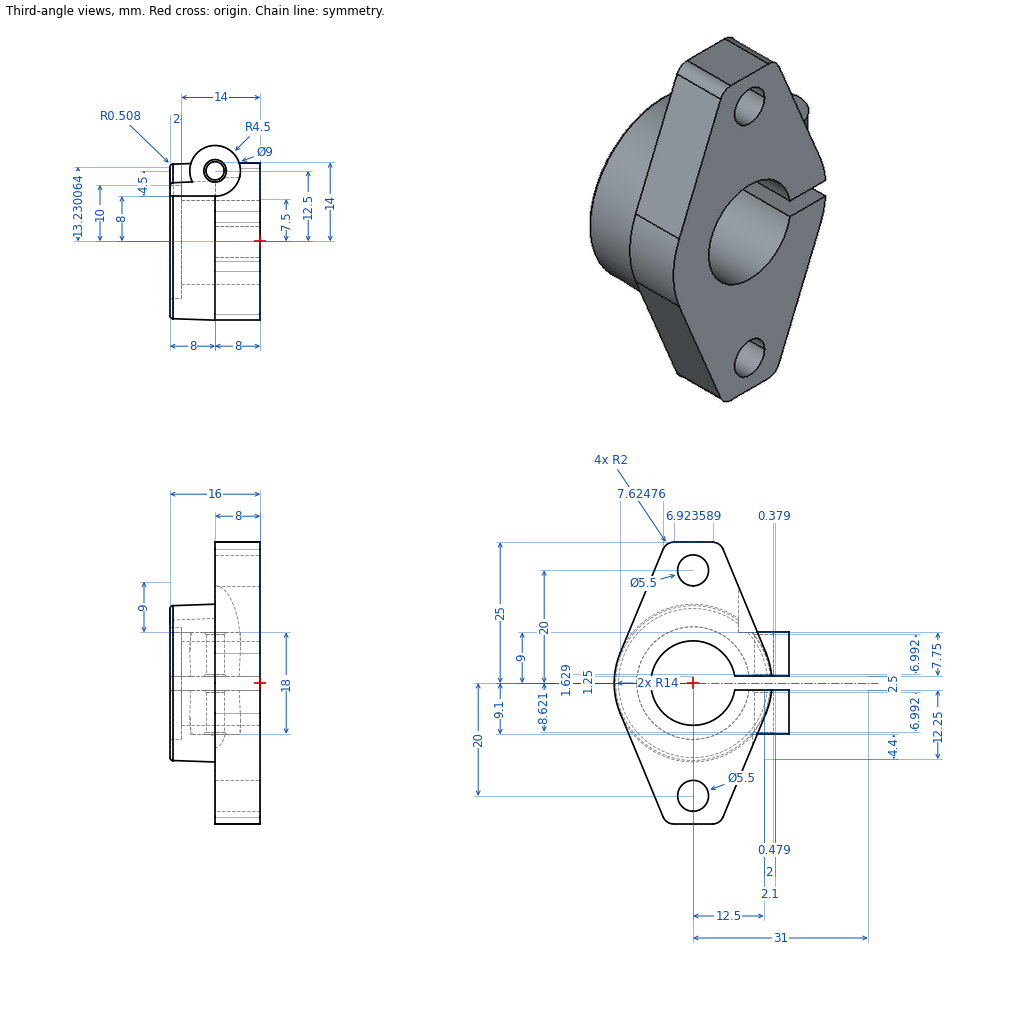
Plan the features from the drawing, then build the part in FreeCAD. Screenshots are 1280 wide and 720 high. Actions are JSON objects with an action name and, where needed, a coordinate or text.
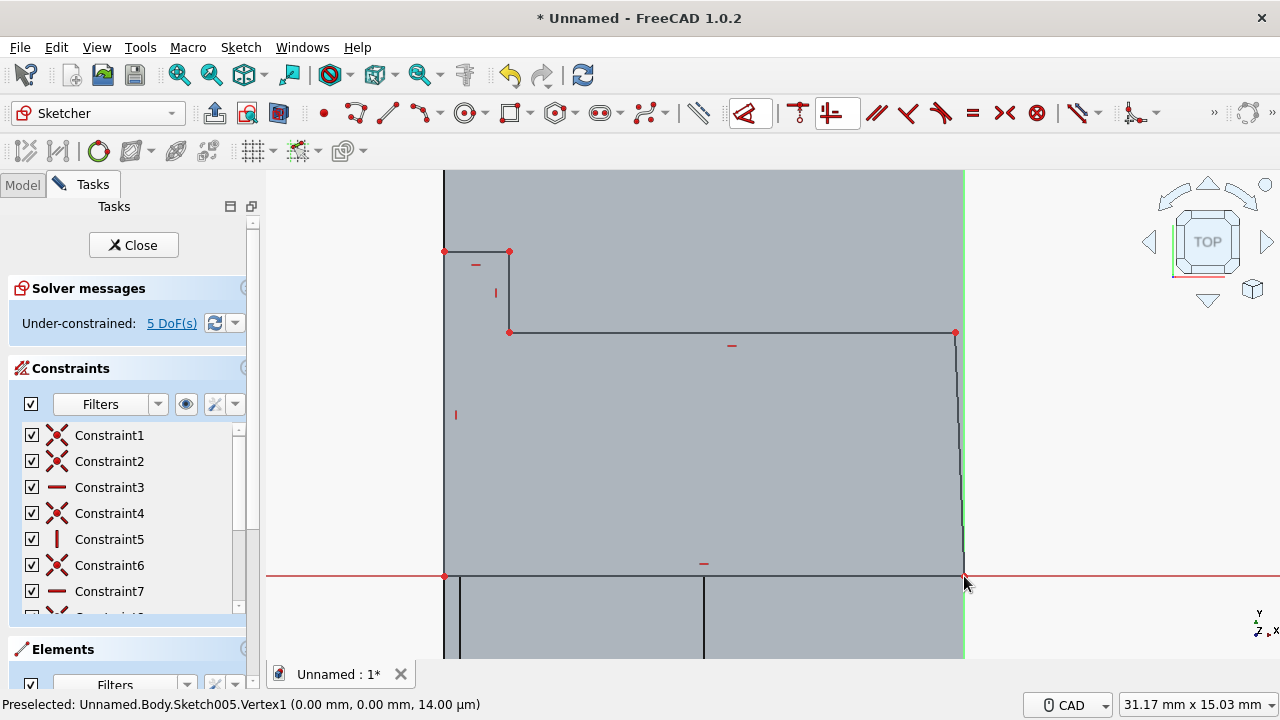
{"action": "left_click", "coordinate": [962, 503]}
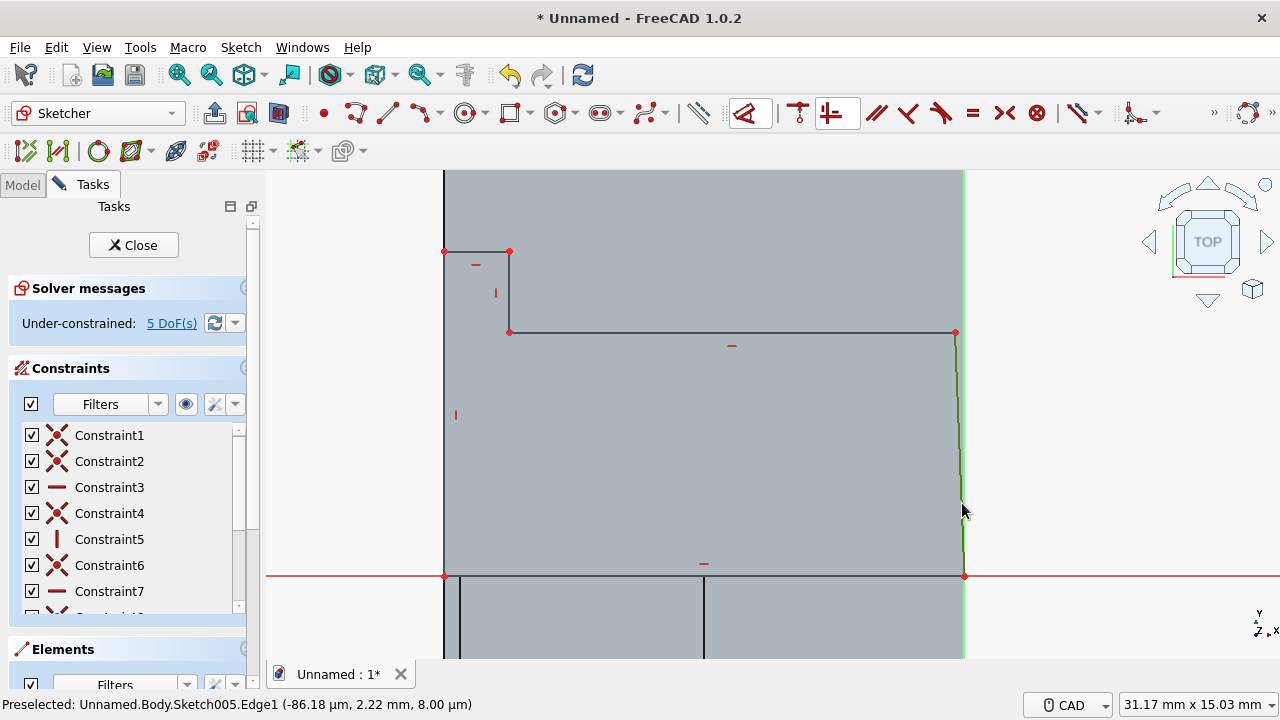
{"action": "left_click", "coordinate": [854, 114]}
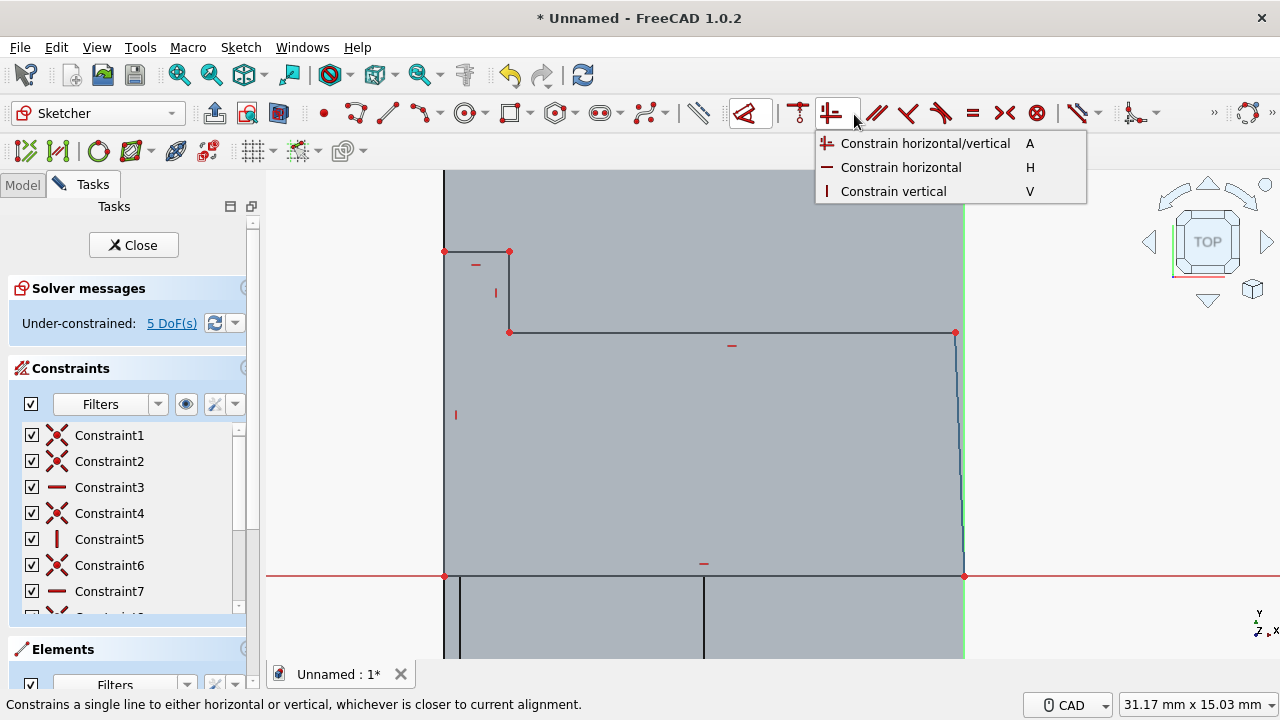
{"action": "left_click", "coordinate": [951, 191]}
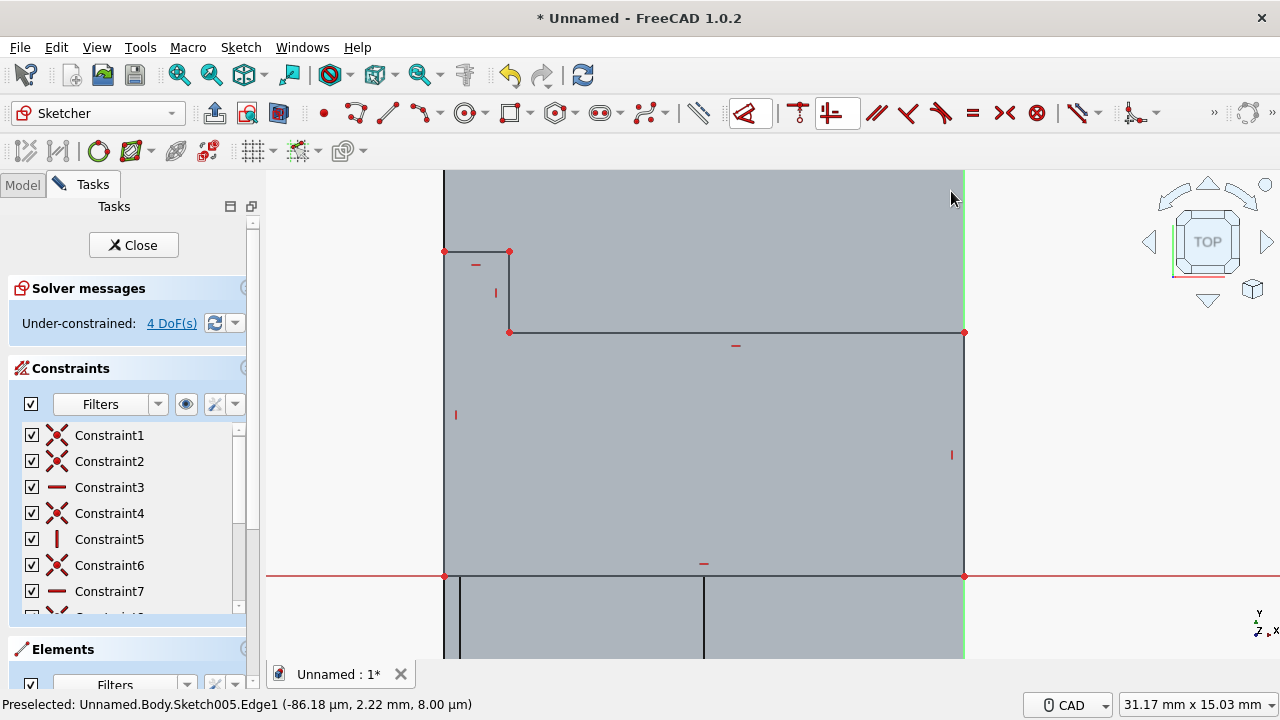
{"action": "left_click", "coordinate": [490, 252]}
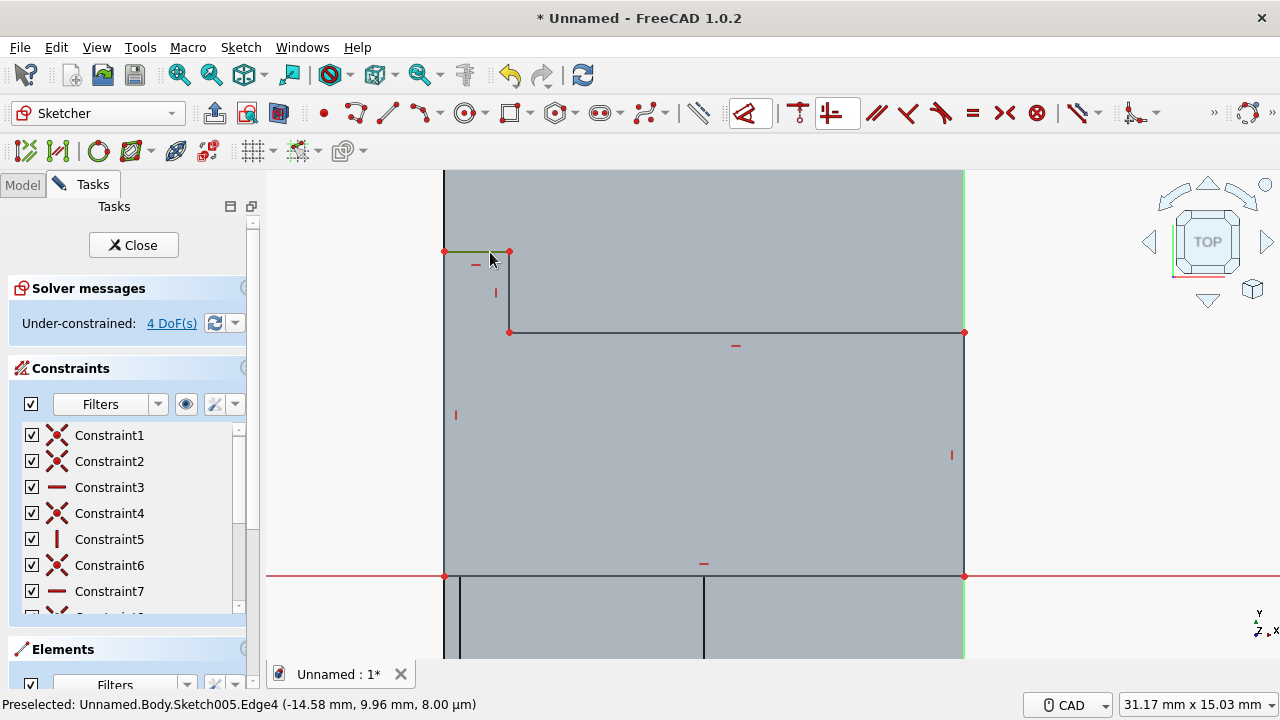
{"action": "key", "text": "l"}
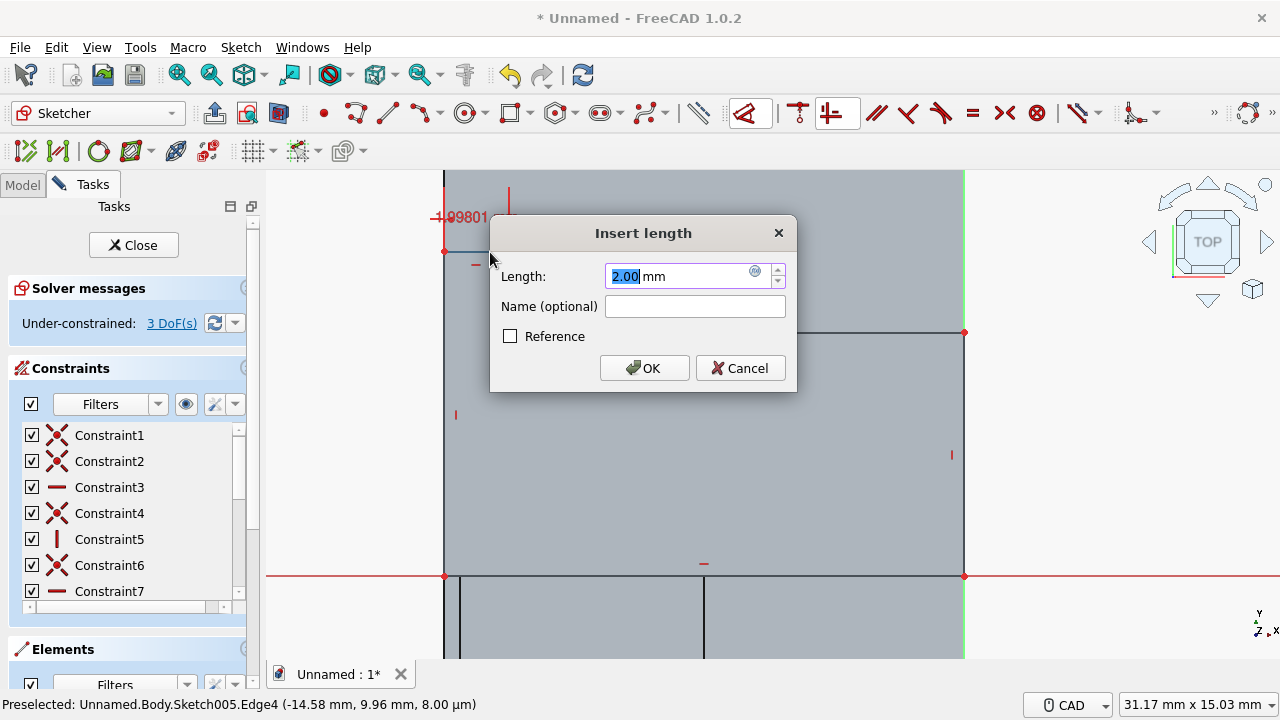
{"action": "type", "text": "2"}
{"action": "key", "text": "Return"}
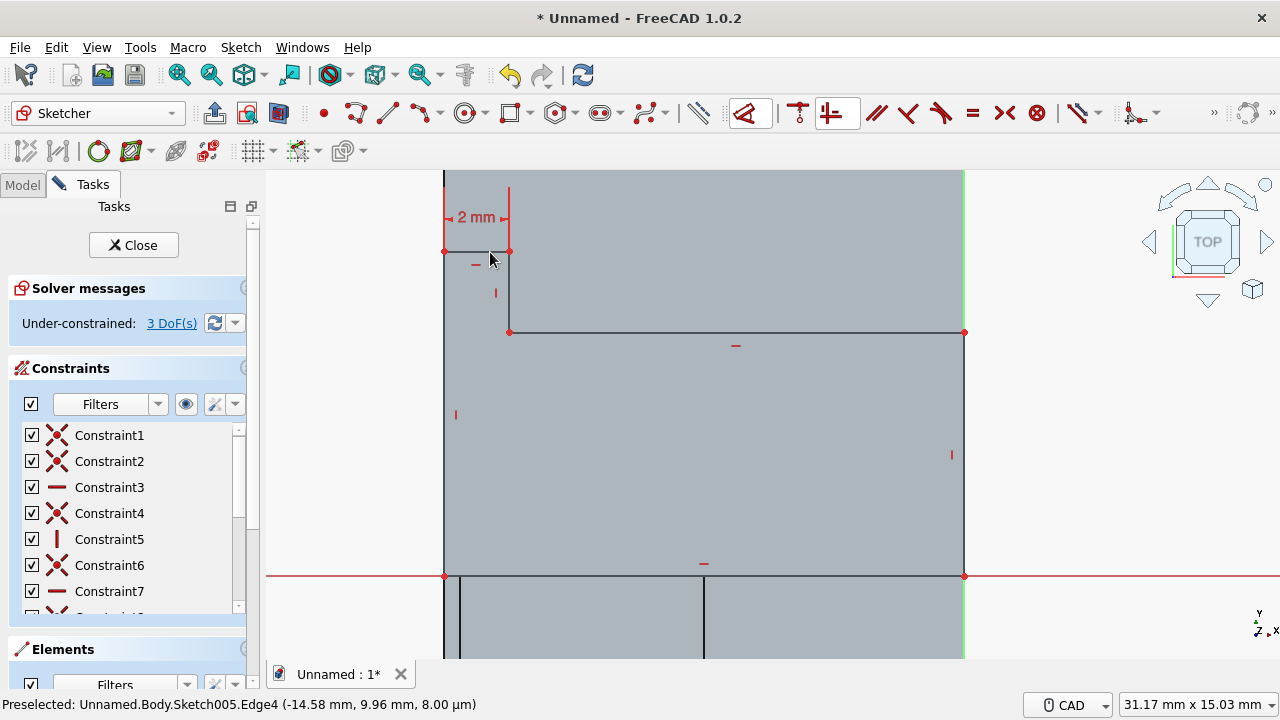
{"action": "left_click", "coordinate": [828, 333]}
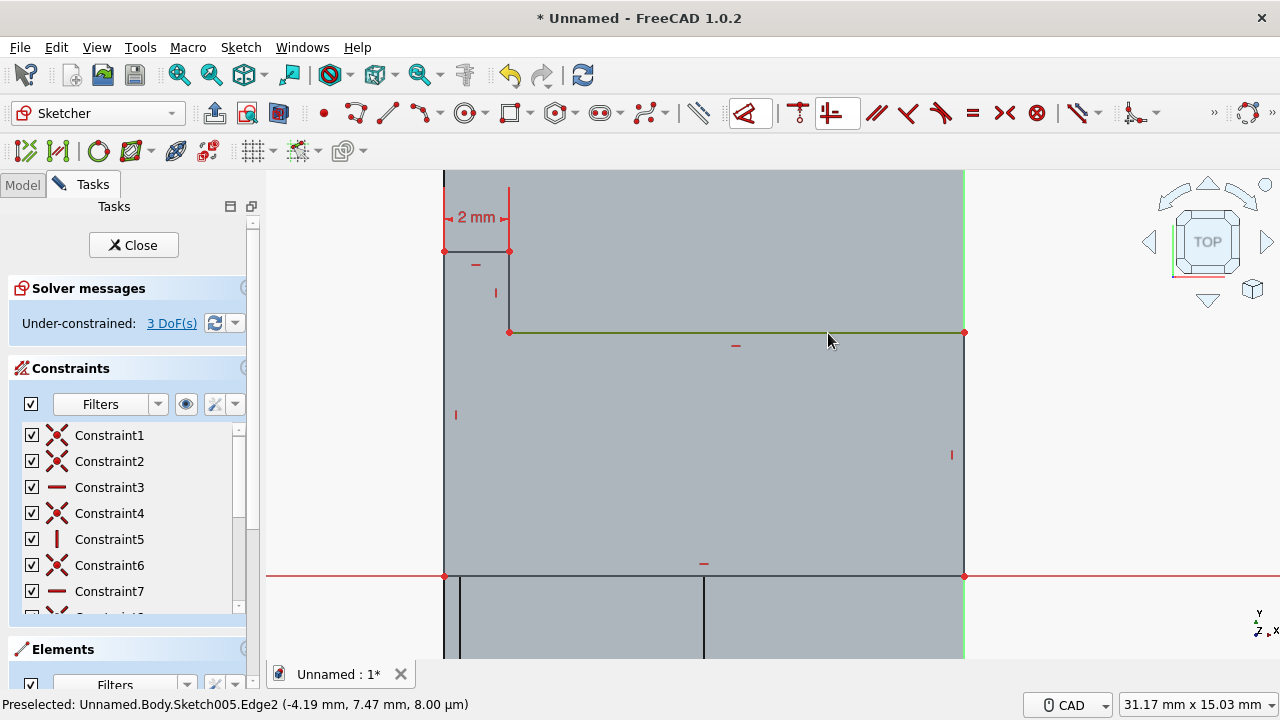
{"action": "key", "text": "l"}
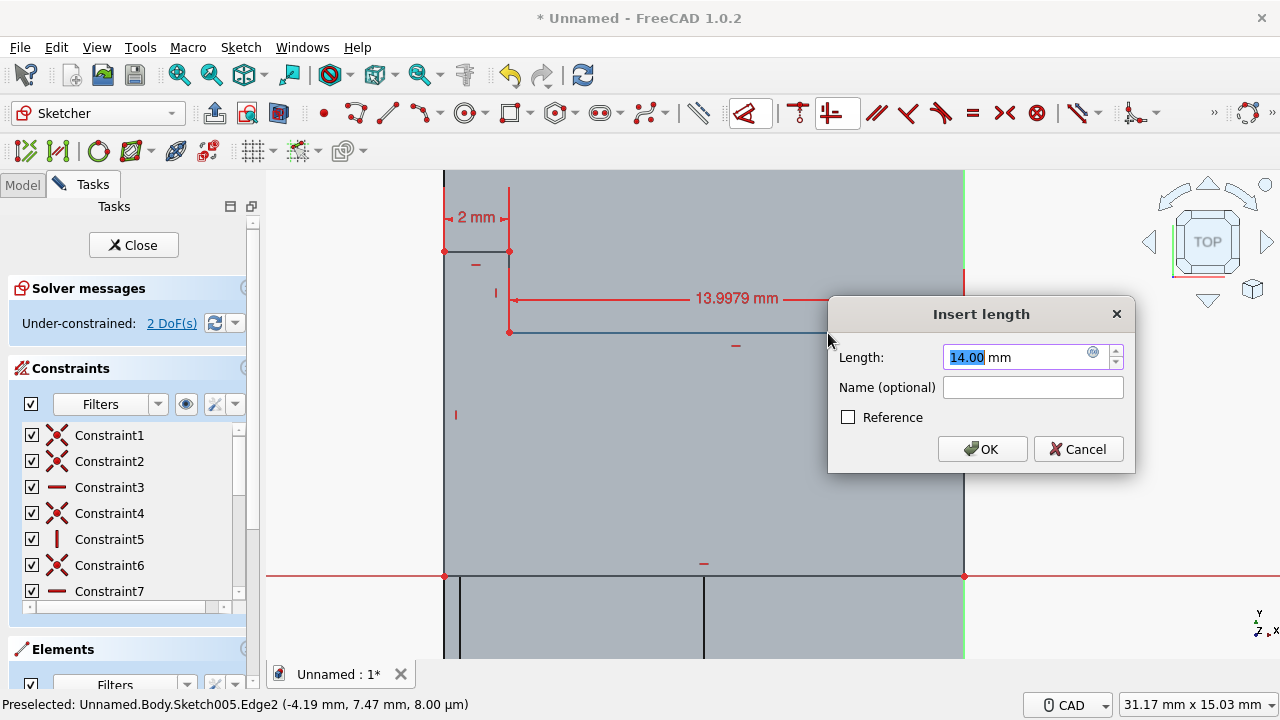
{"action": "type", "text": "14"}
{"action": "key", "text": "Return"}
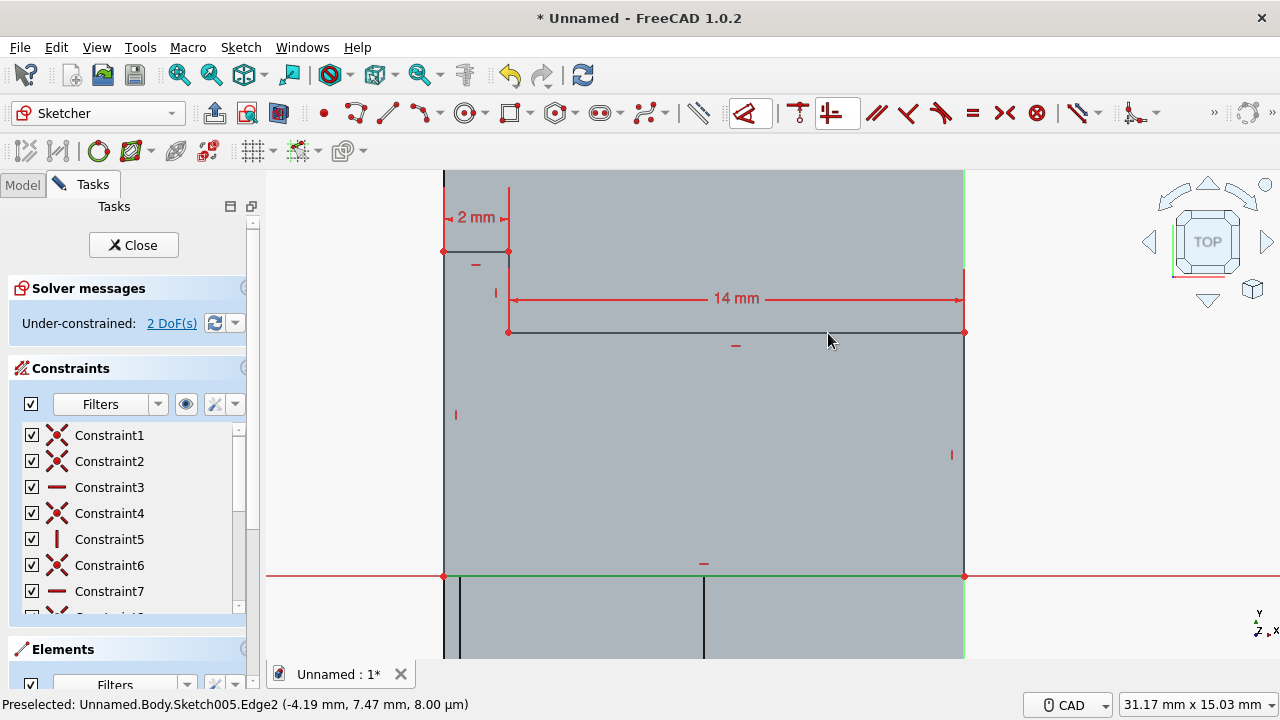
{"action": "left_click", "coordinate": [444, 349]}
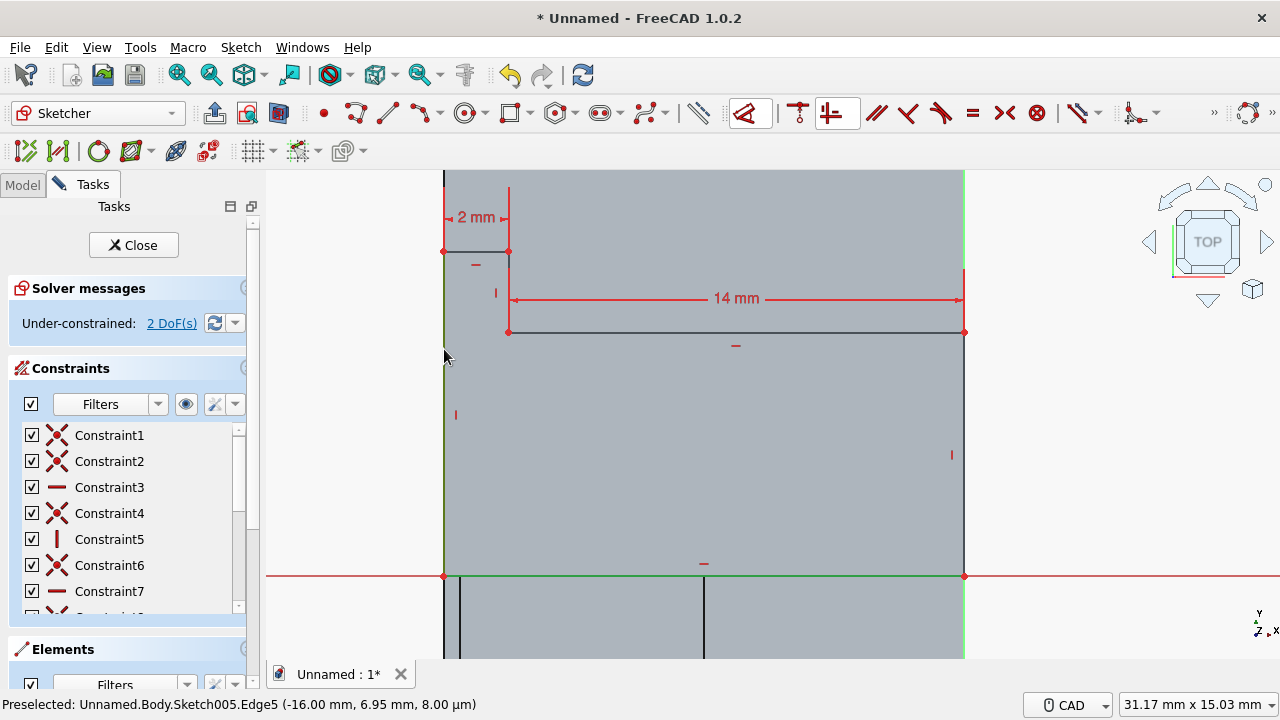
{"action": "left_click", "coordinate": [766, 114]}